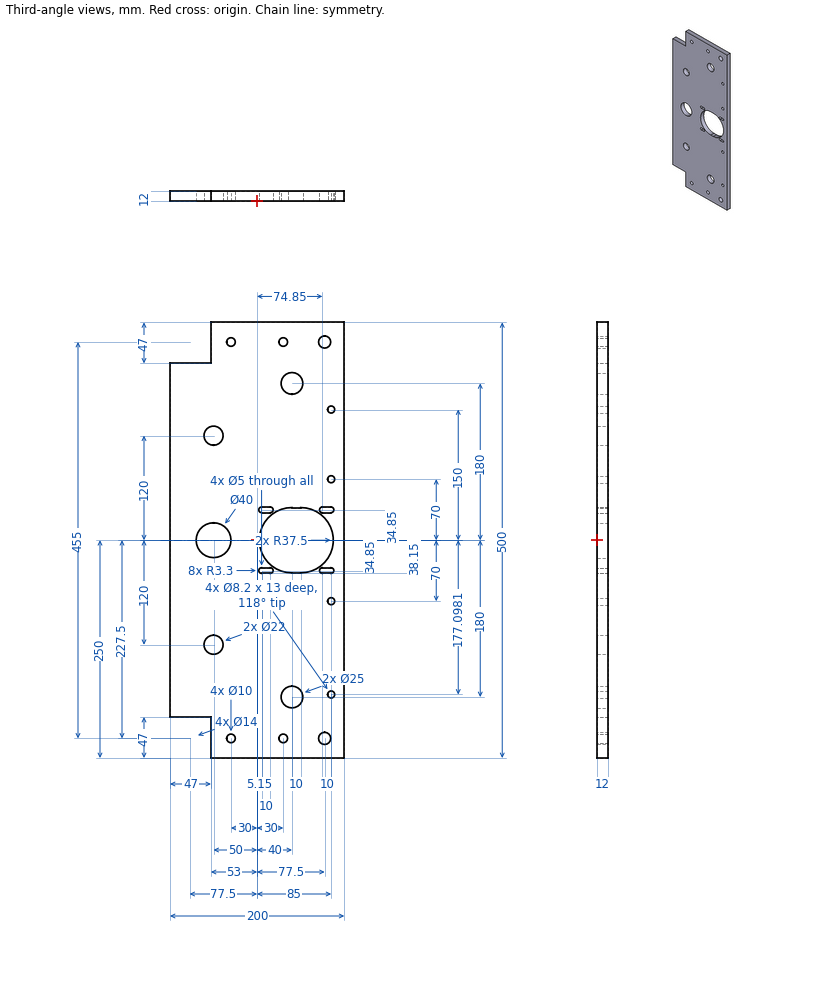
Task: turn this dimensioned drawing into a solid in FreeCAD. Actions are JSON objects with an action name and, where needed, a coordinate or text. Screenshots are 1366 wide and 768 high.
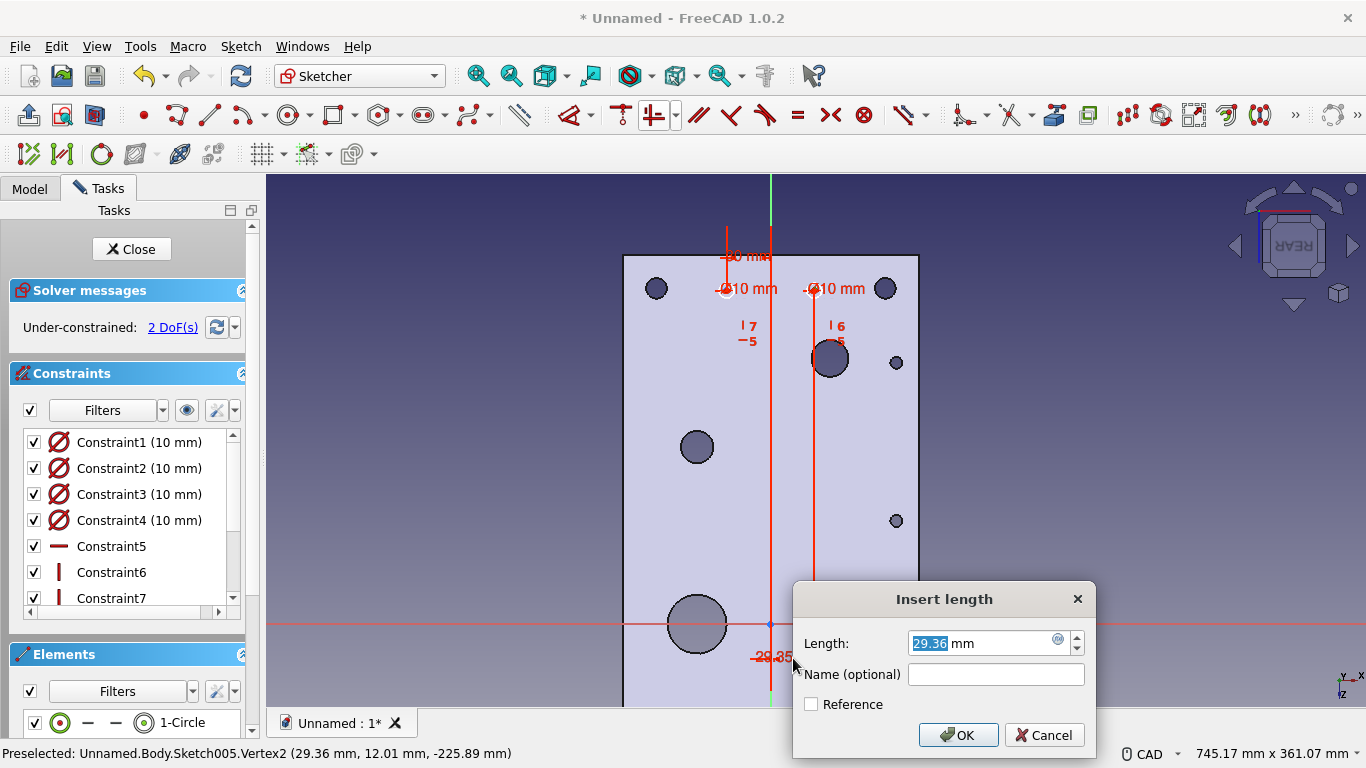
{"action": "type", "text": "30"}
{"action": "key", "text": "Return"}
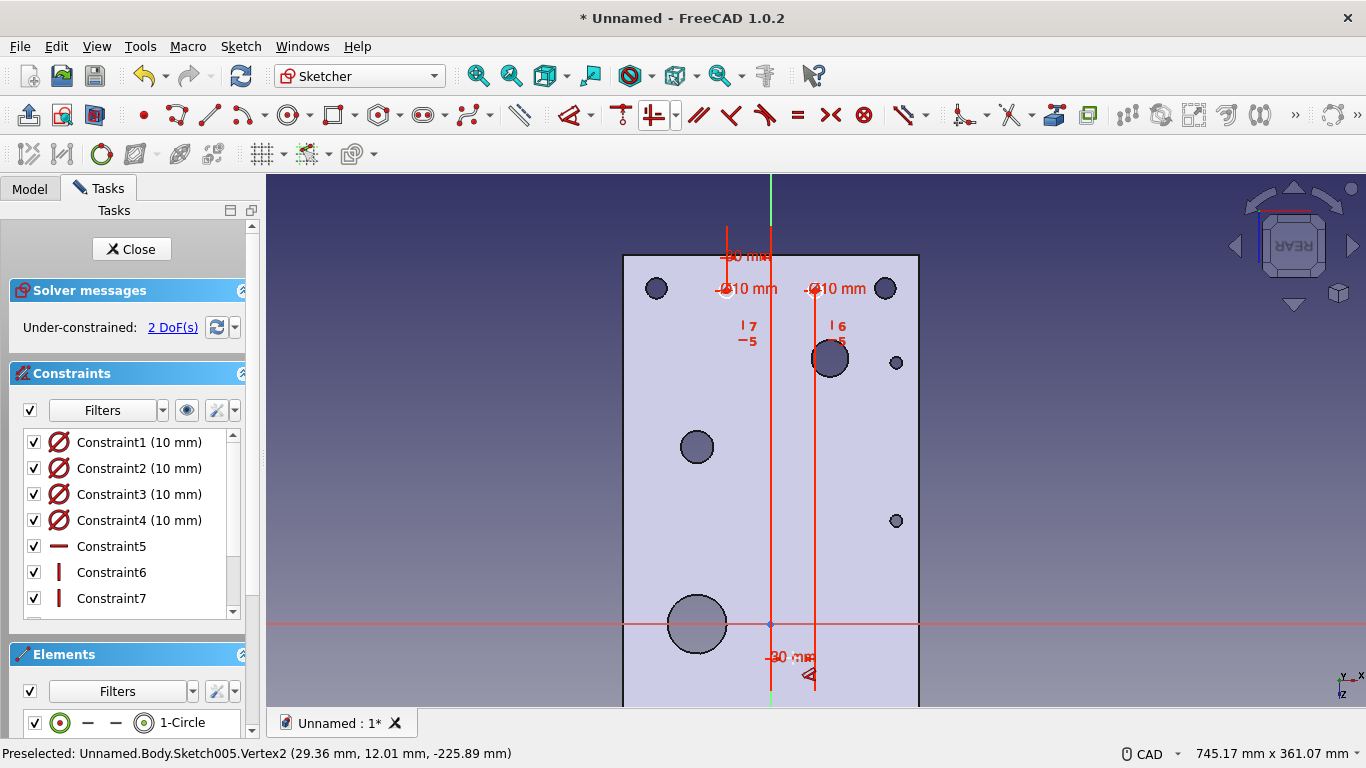
{"action": "left_click", "coordinate": [815, 291]}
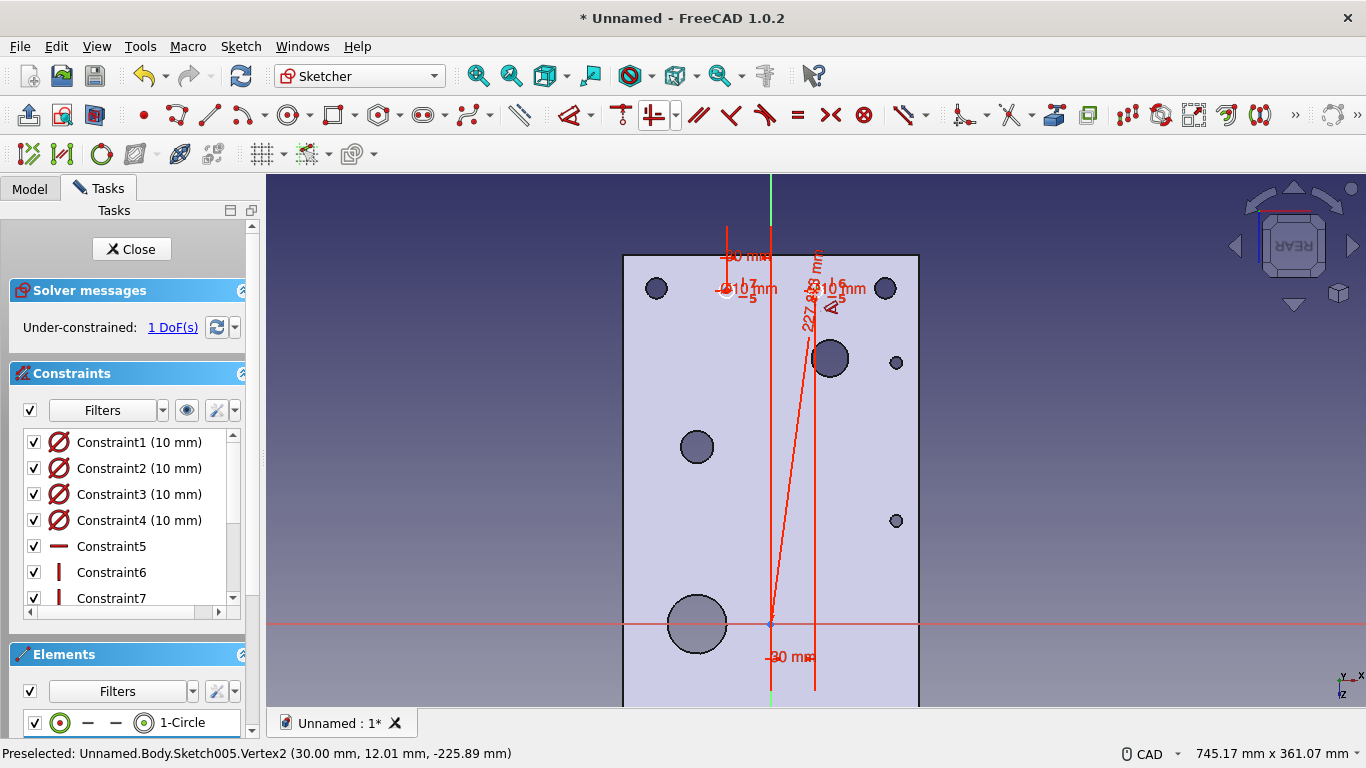
{"action": "scroll", "coordinate": [728, 291], "scroll_direction": "down", "scroll_amount": 4}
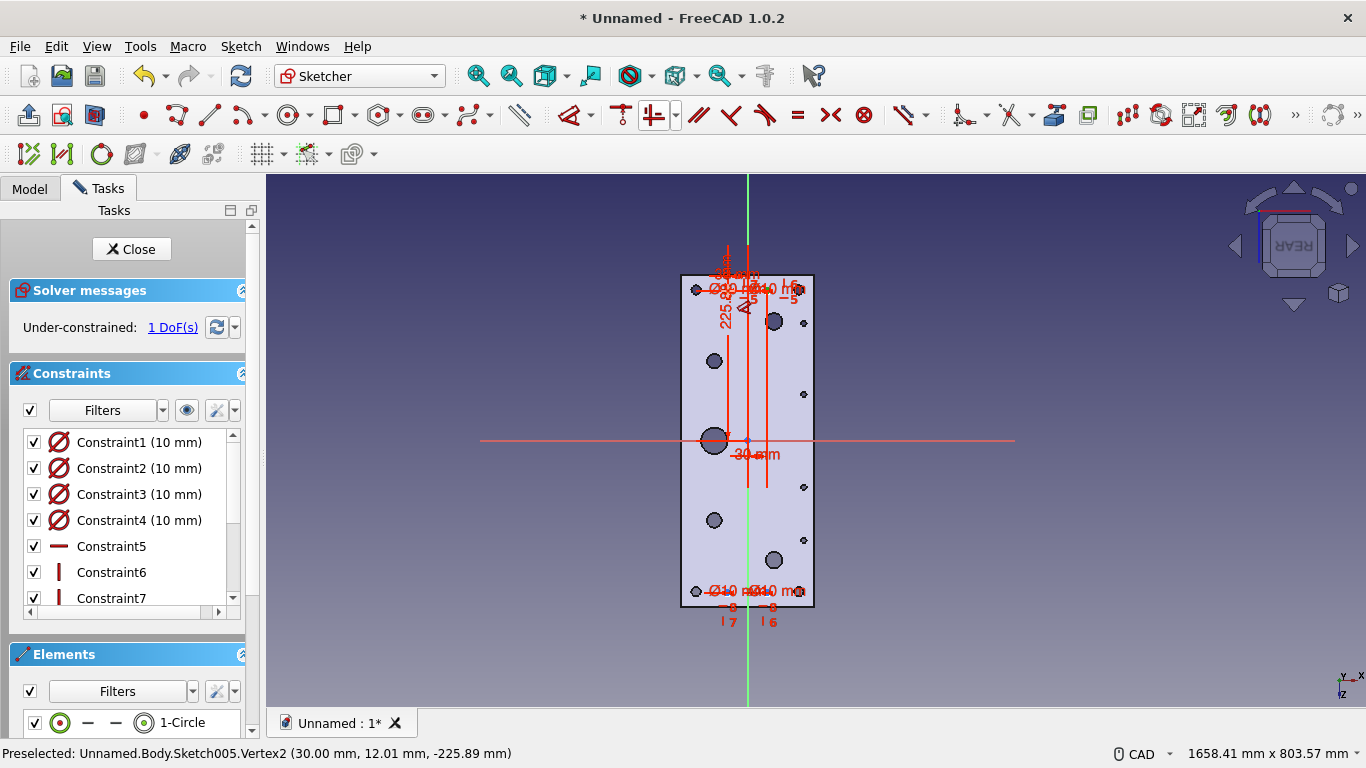
{"action": "left_click", "coordinate": [767, 593]}
{"action": "left_click", "coordinate": [801, 373]}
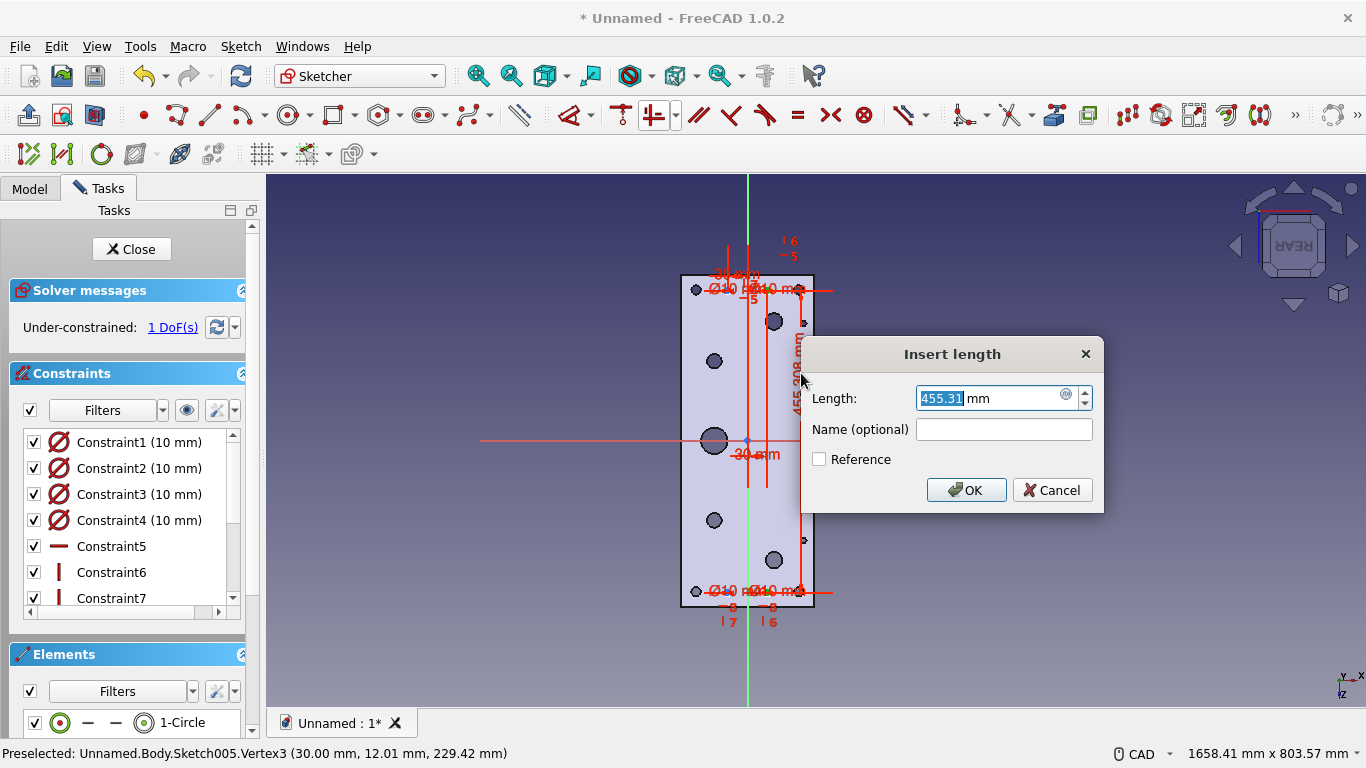
{"action": "type", "text": "455"}
{"action": "key", "text": "Return"}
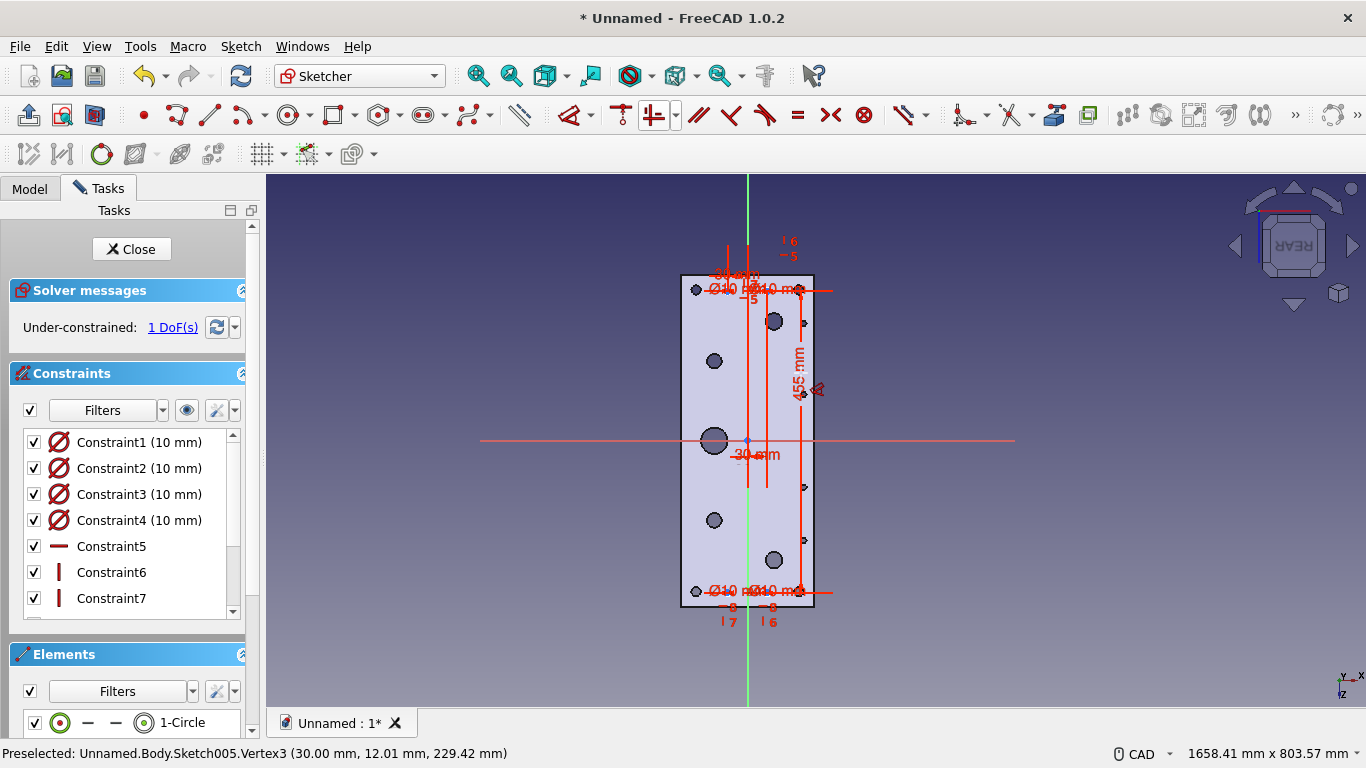
{"action": "left_click", "coordinate": [728, 291]}
{"action": "left_click", "coordinate": [694, 366]}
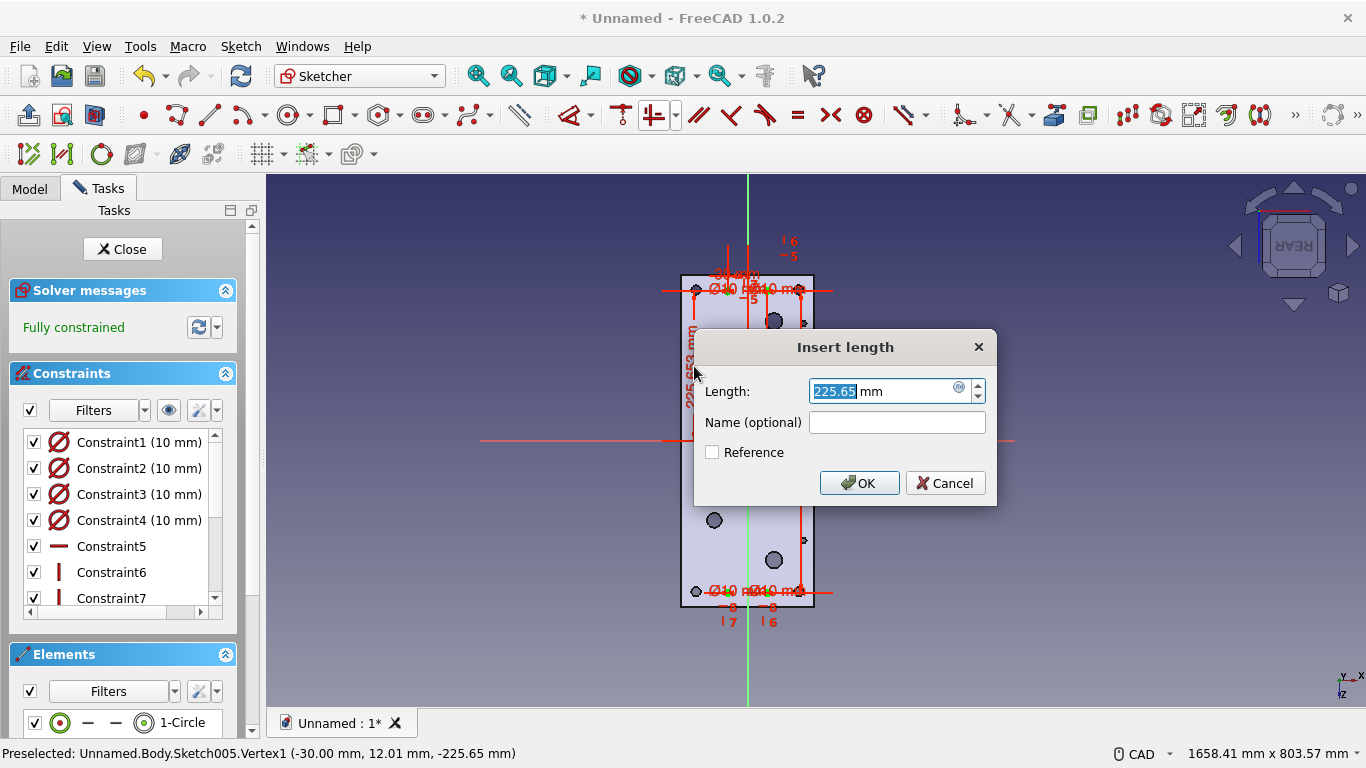
{"action": "type", "text": "227.5"}
{"action": "key", "text": "Return"}
{"action": "key", "text": "Escape"}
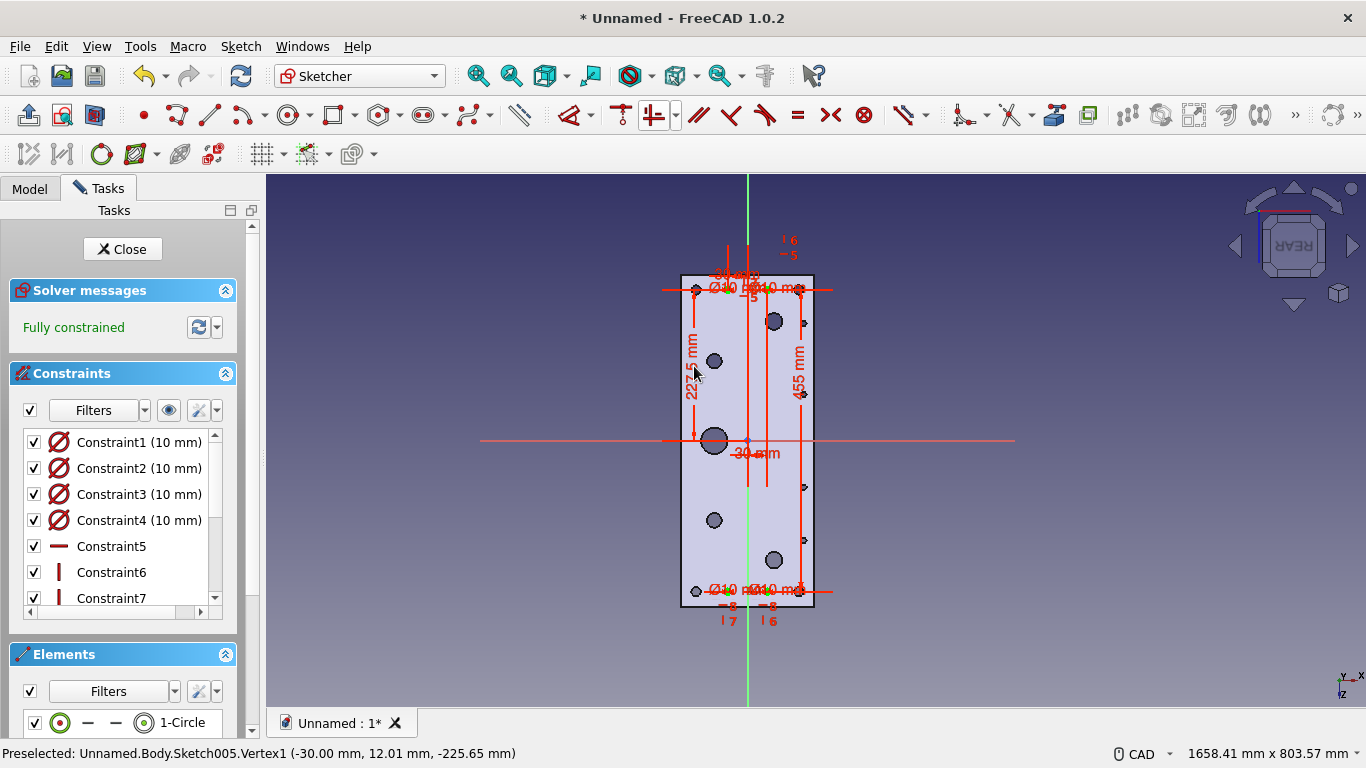
{"action": "left_click", "coordinate": [123, 249]}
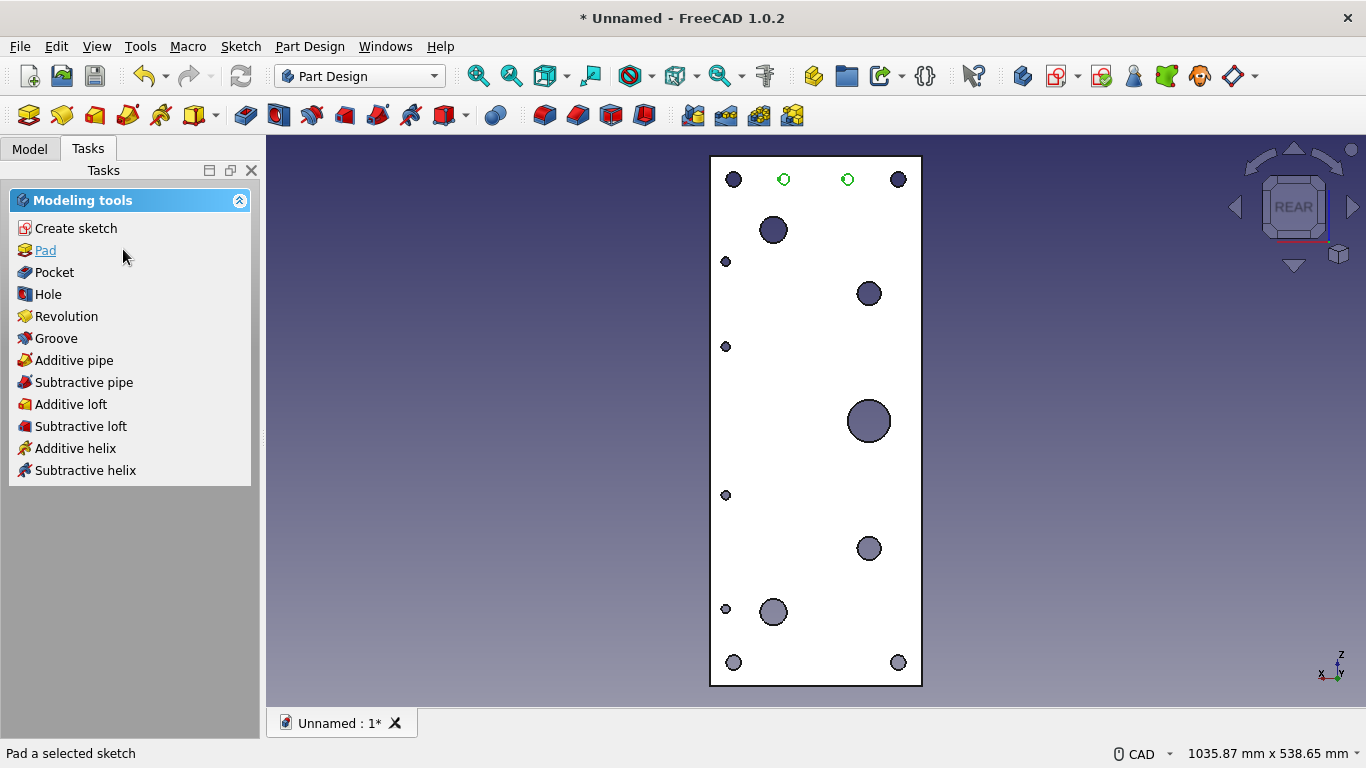
{"action": "left_click", "coordinate": [246, 116]}